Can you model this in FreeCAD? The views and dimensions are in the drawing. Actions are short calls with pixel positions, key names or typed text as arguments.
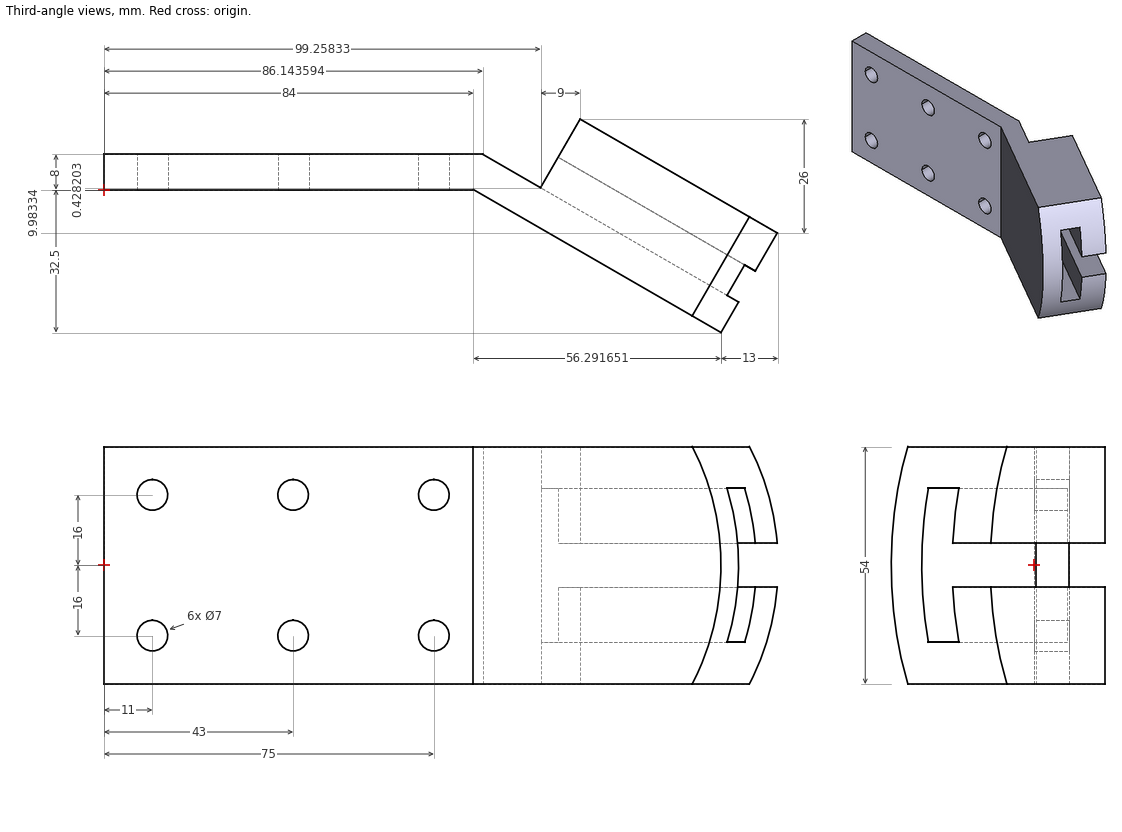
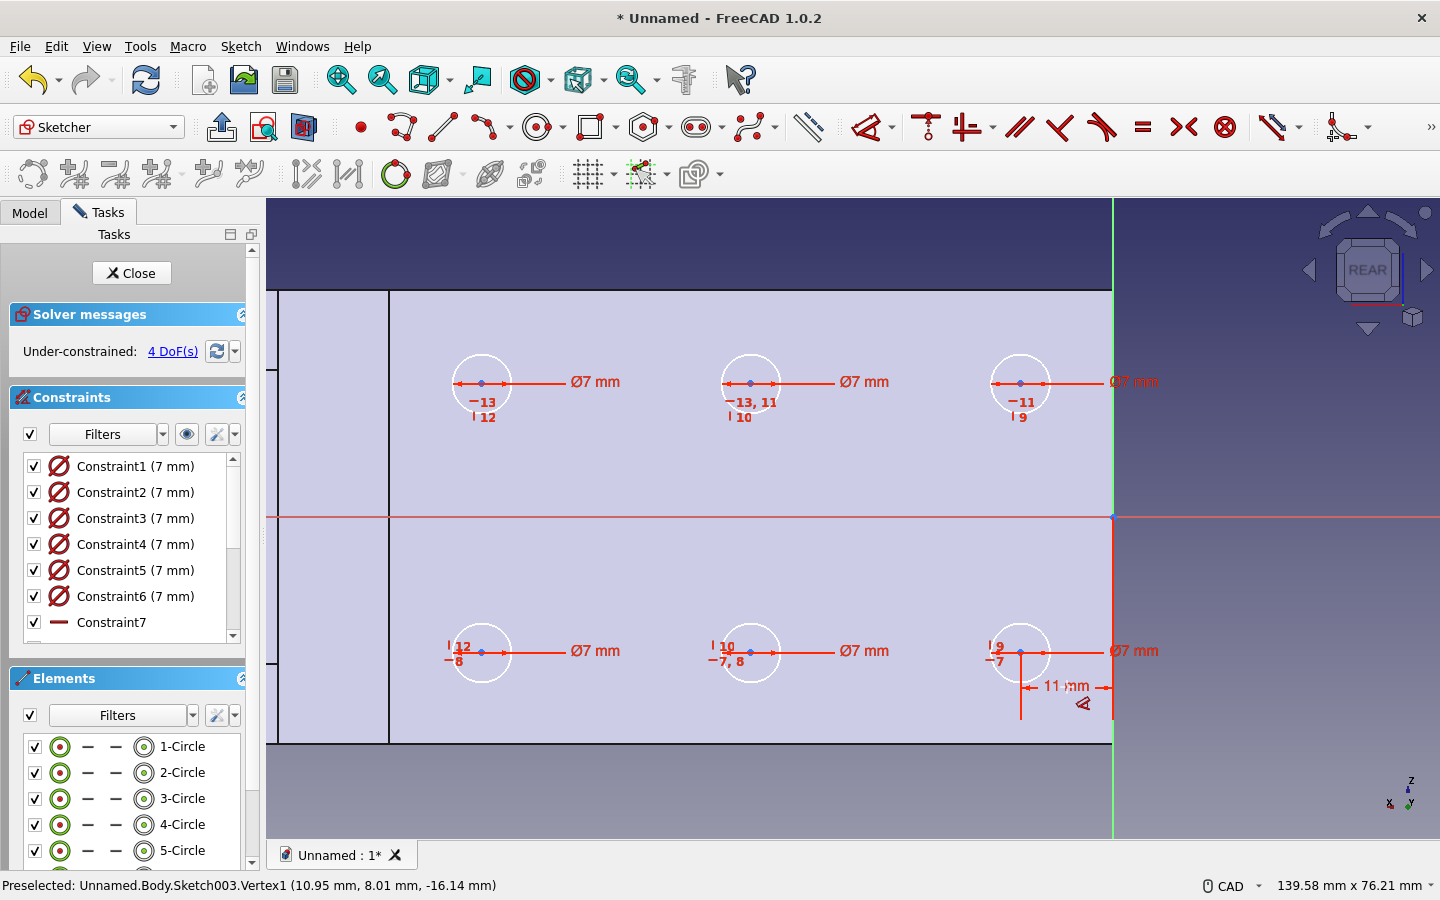
click(1021, 653)
click(1147, 585)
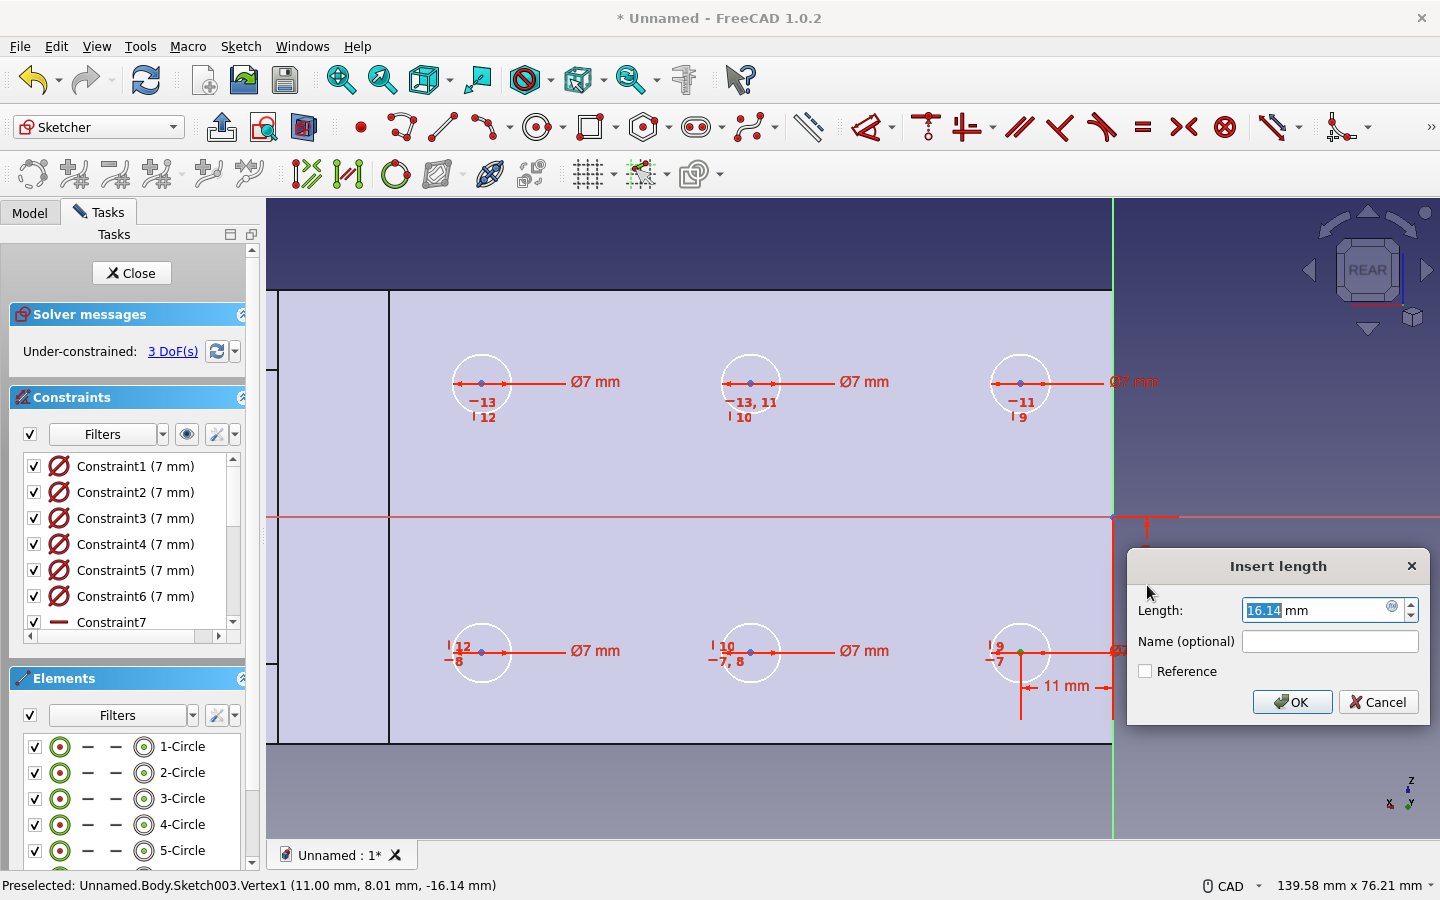
text(16)
key(Return)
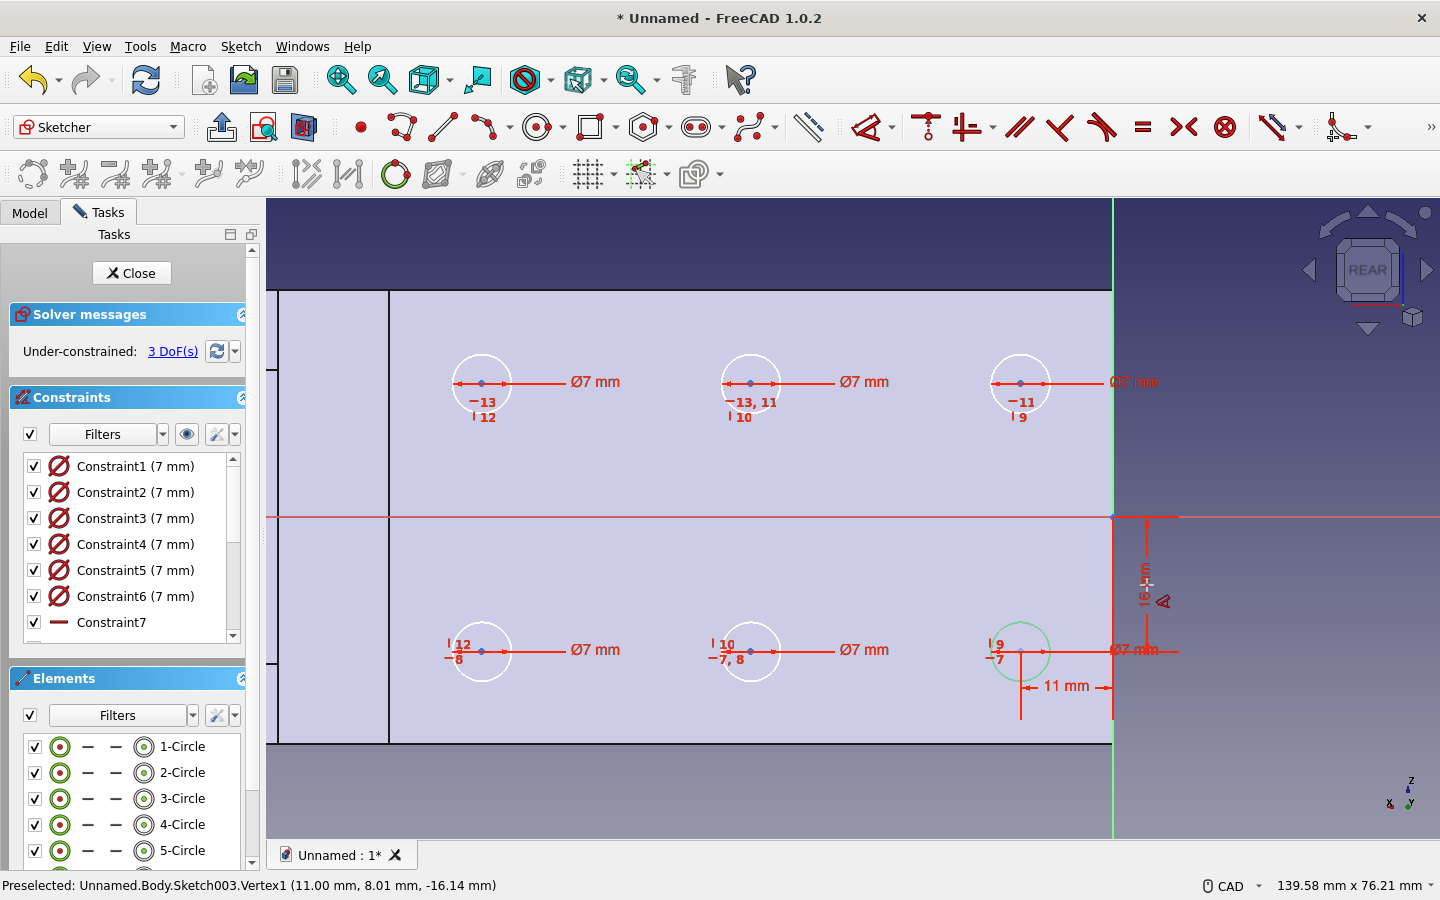
click(751, 652)
click(932, 686)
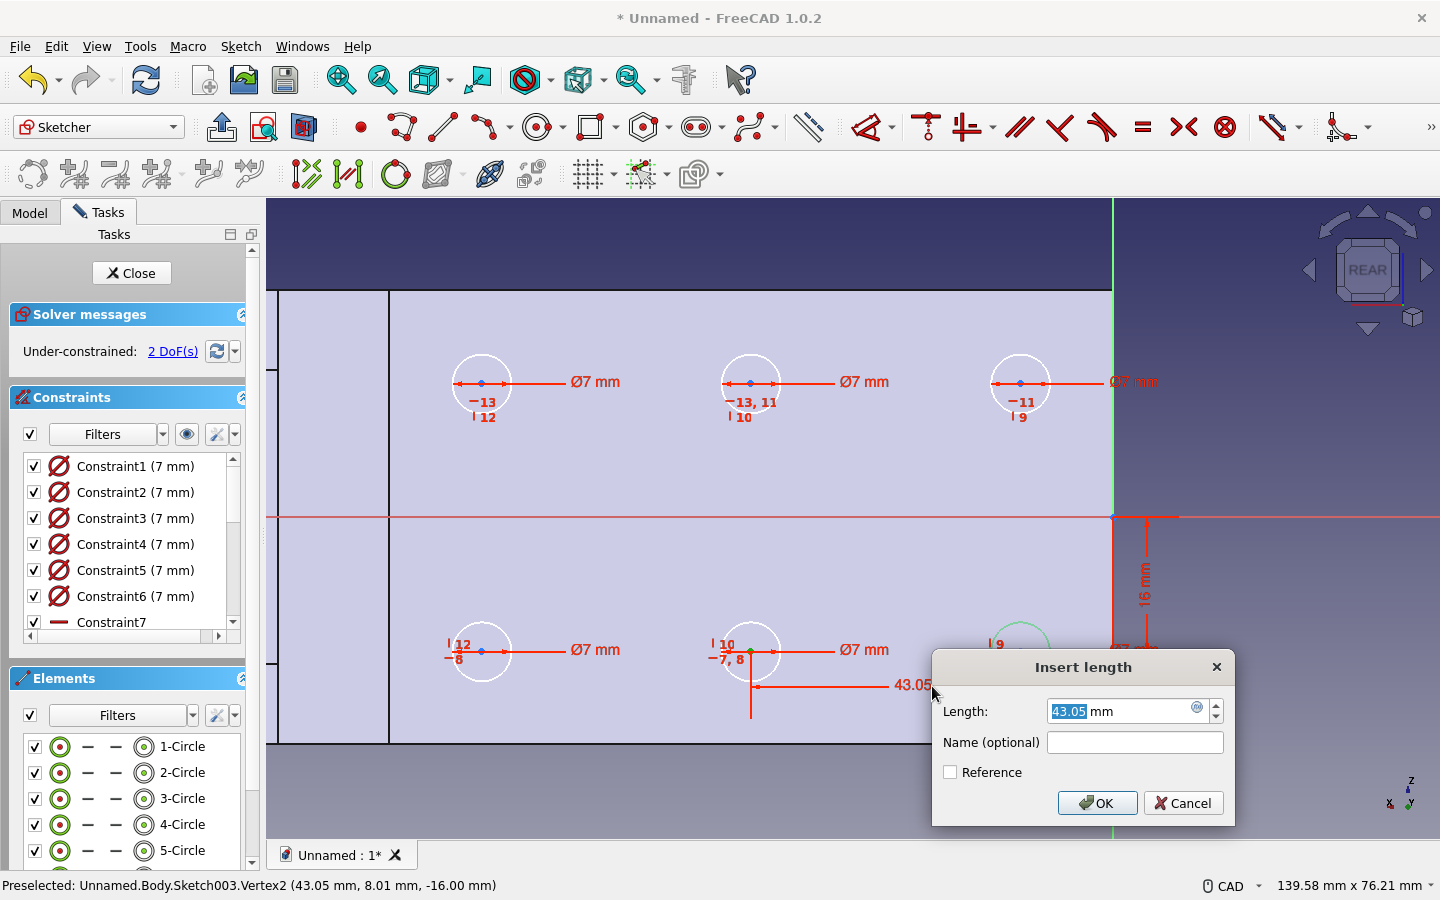
text(43)
key(Return)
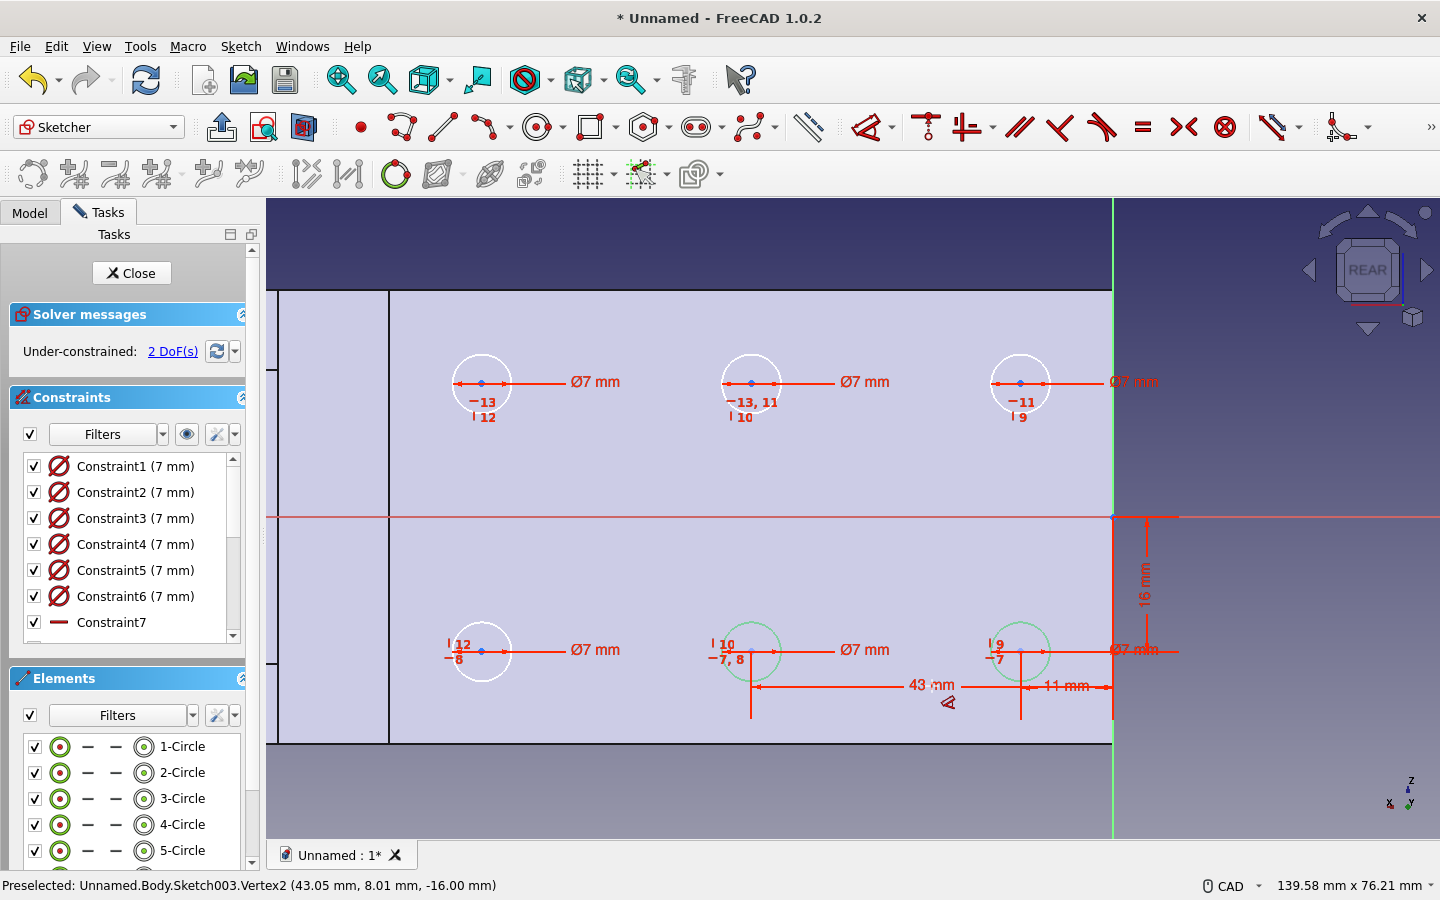
click(482, 652)
click(798, 686)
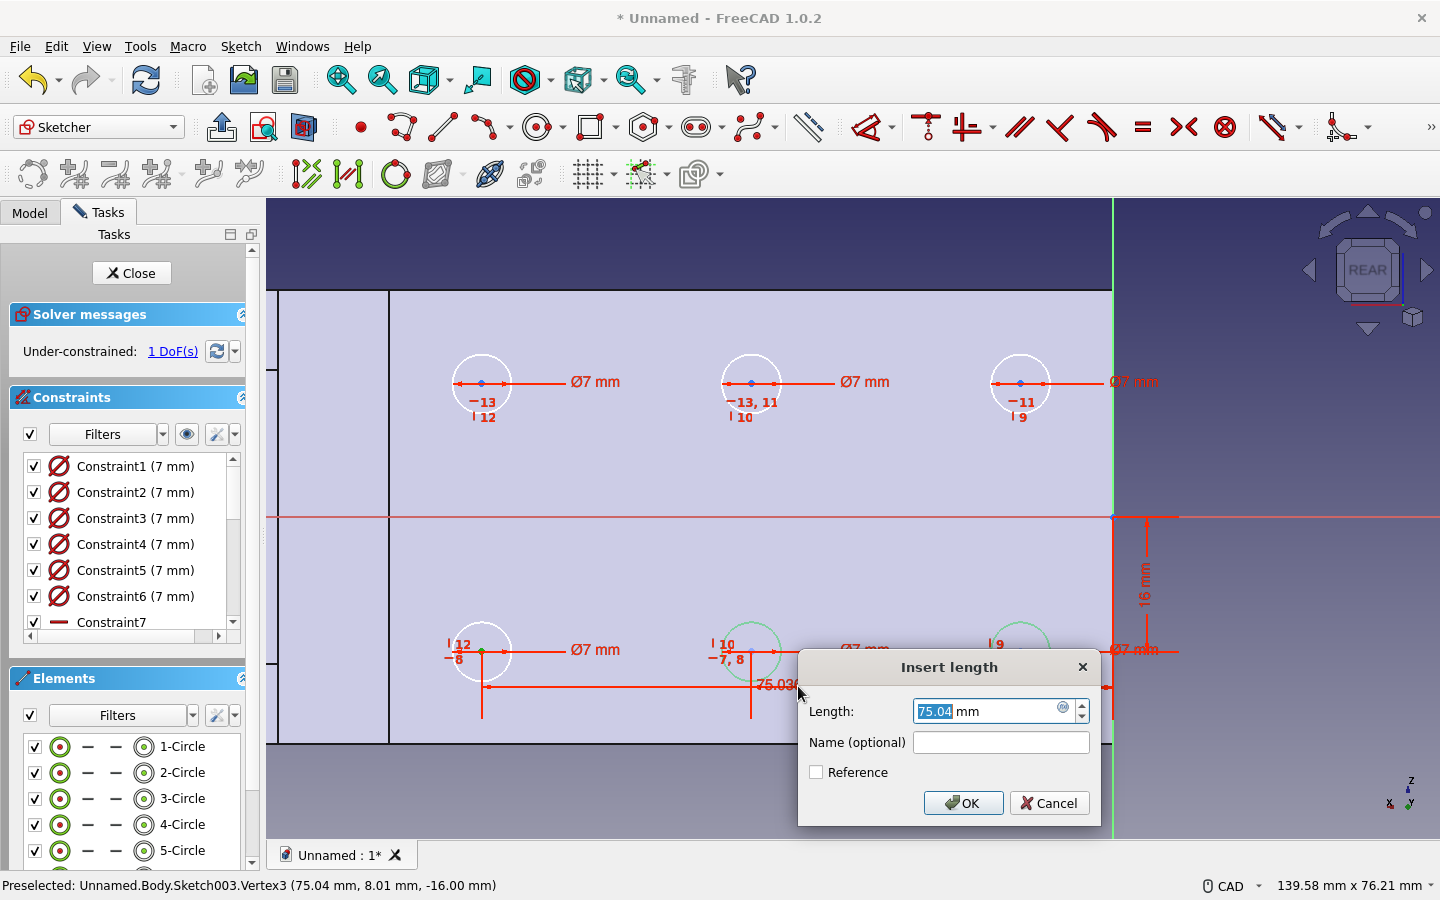
text(75)
key(Return)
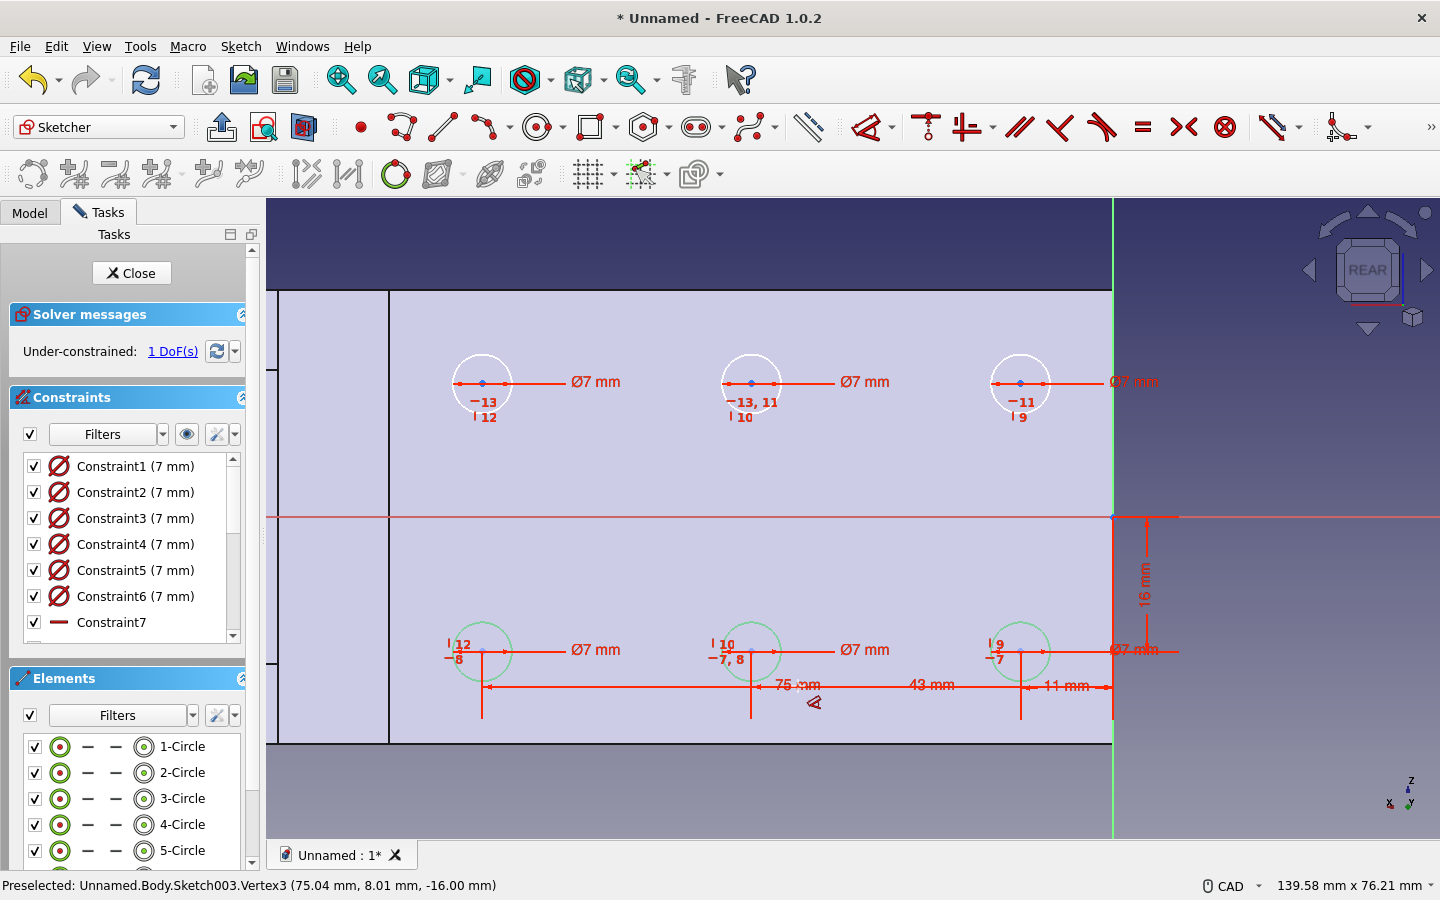
click(1021, 384)
click(1147, 451)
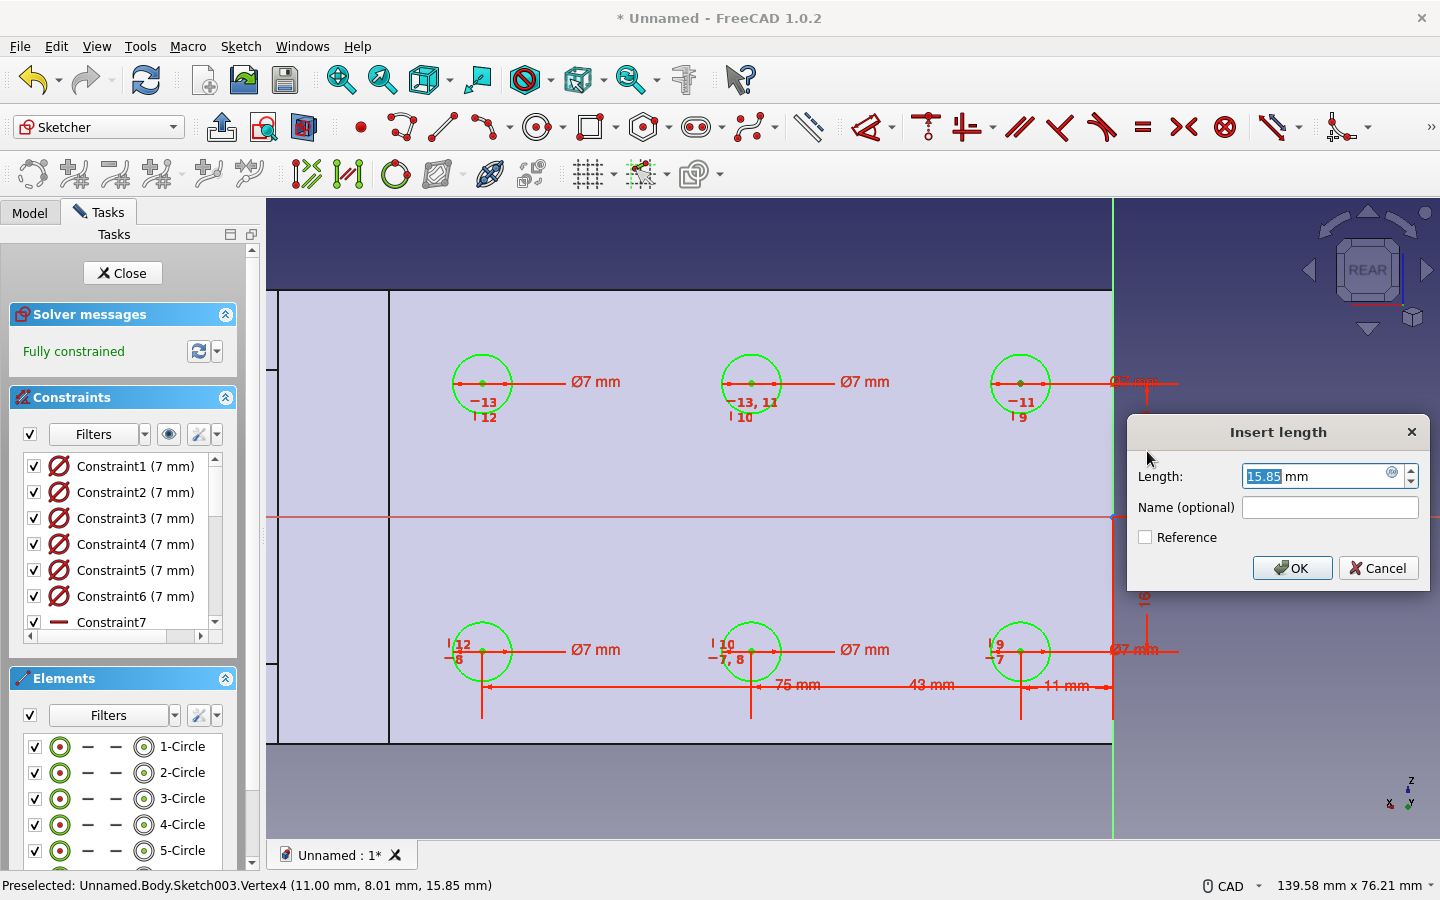
text(16)
key(Return)
key(Escape)